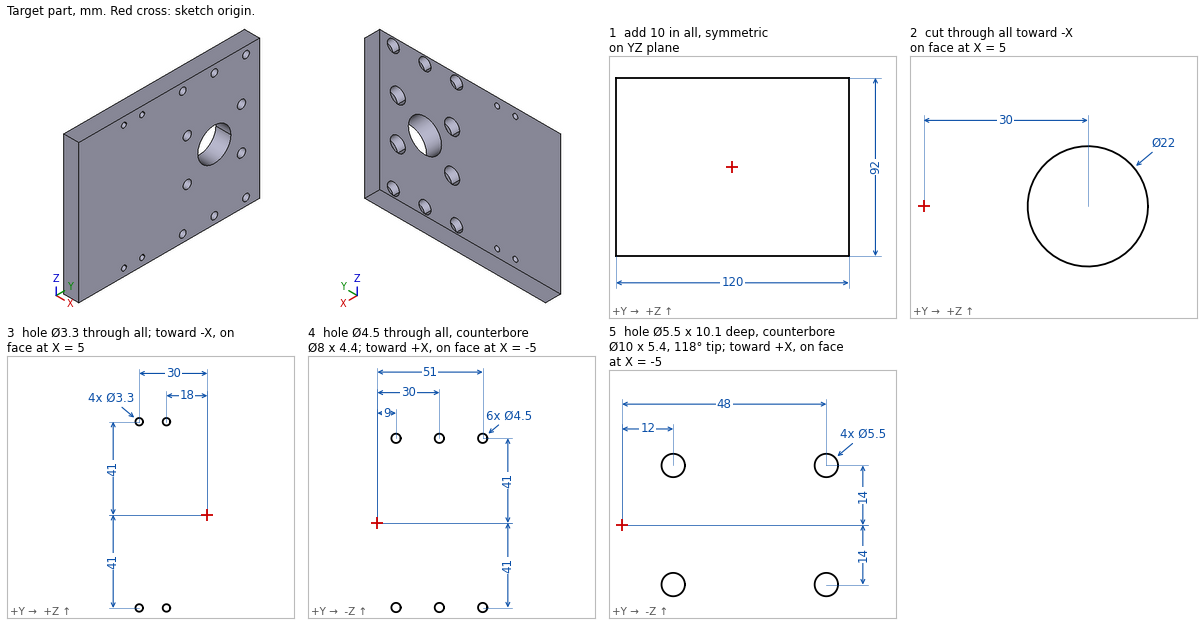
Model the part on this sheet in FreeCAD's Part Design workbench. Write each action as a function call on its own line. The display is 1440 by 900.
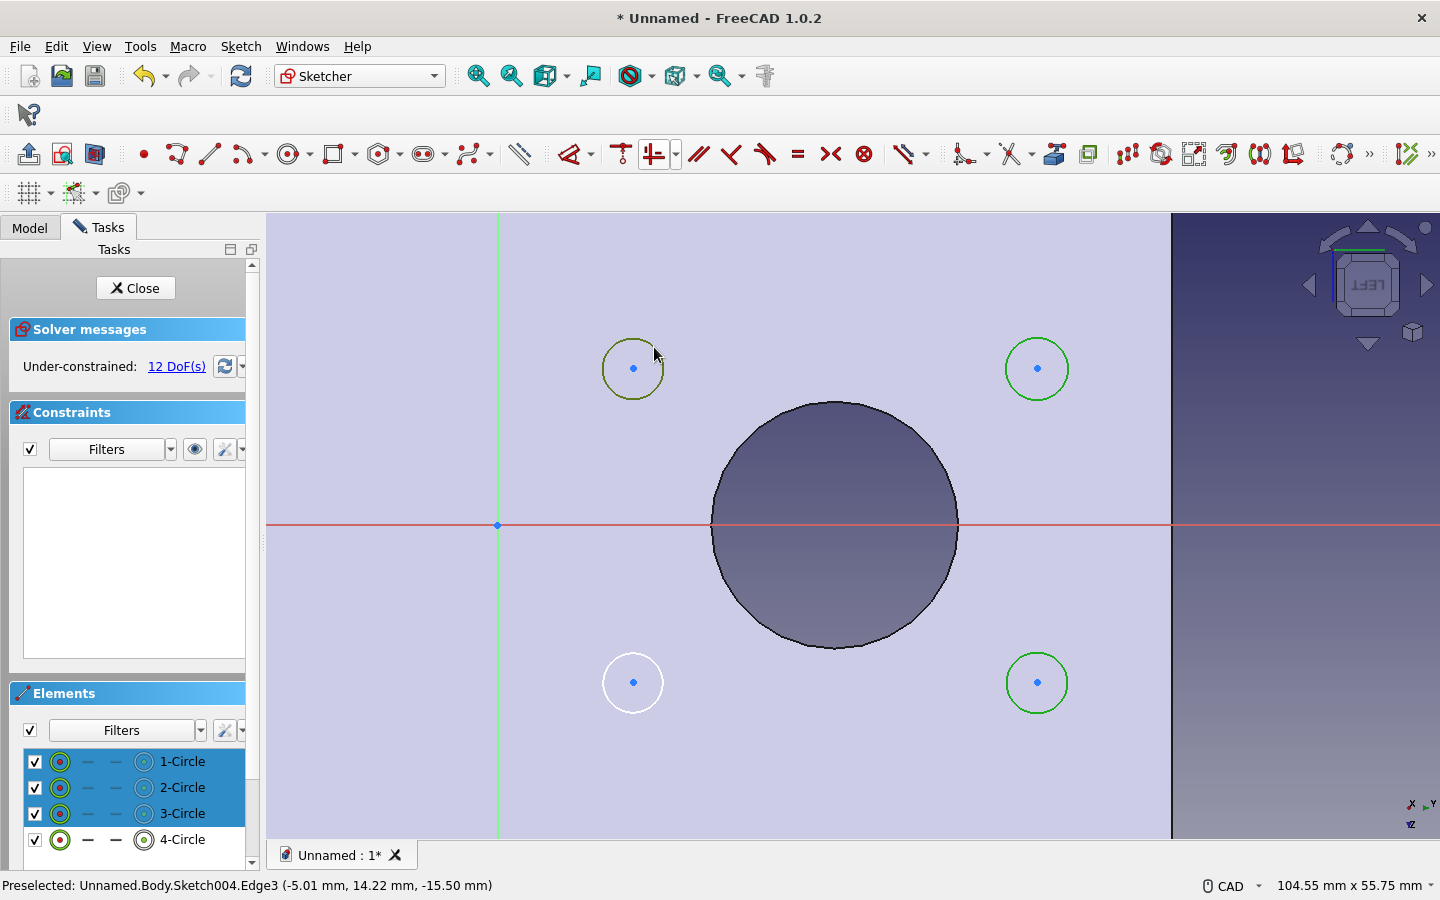
click(654, 662)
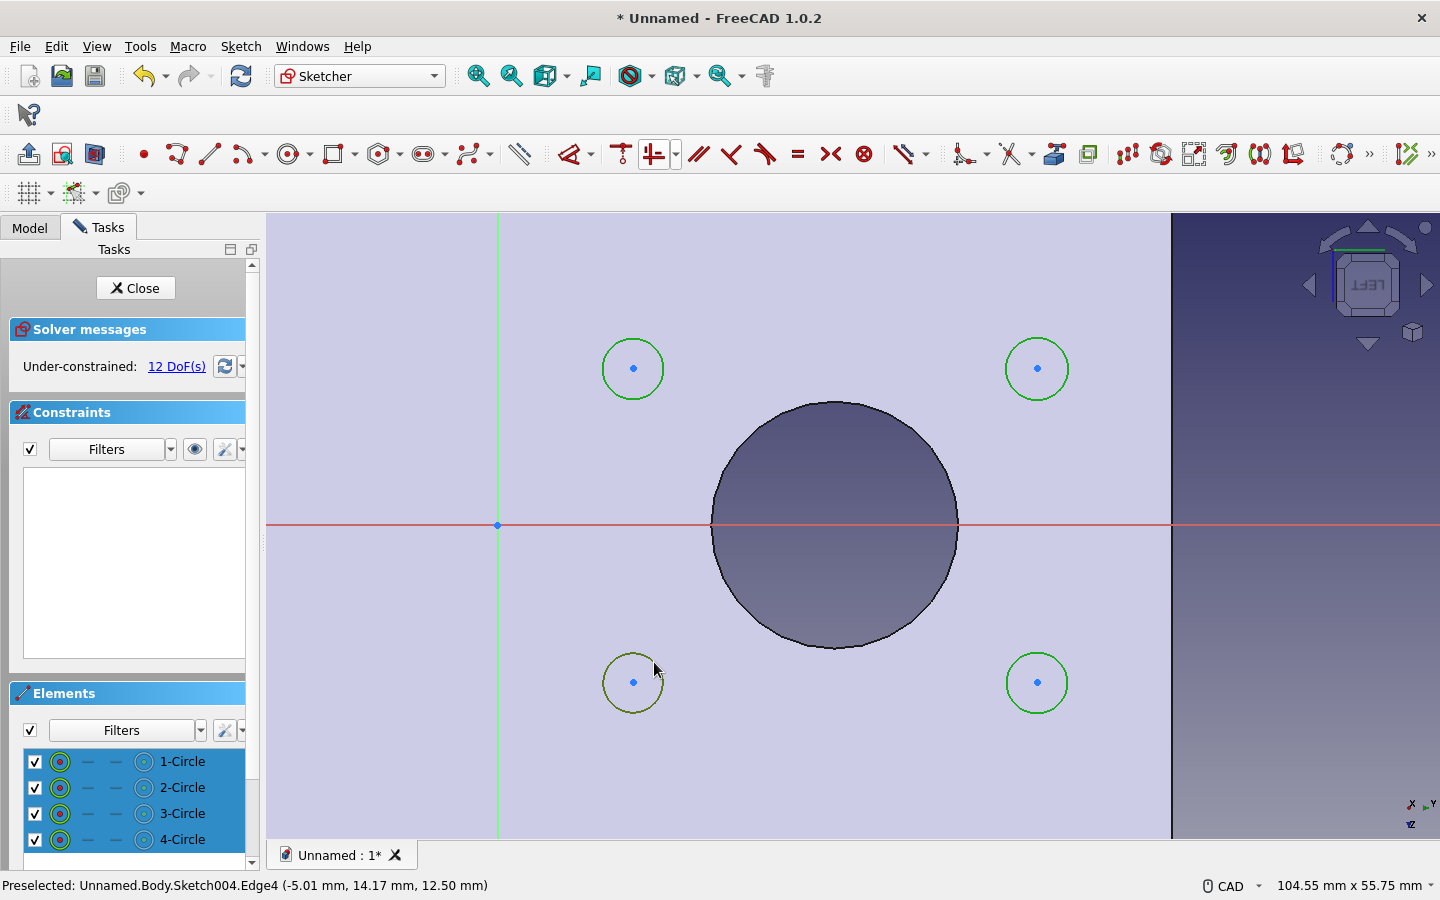
key(e)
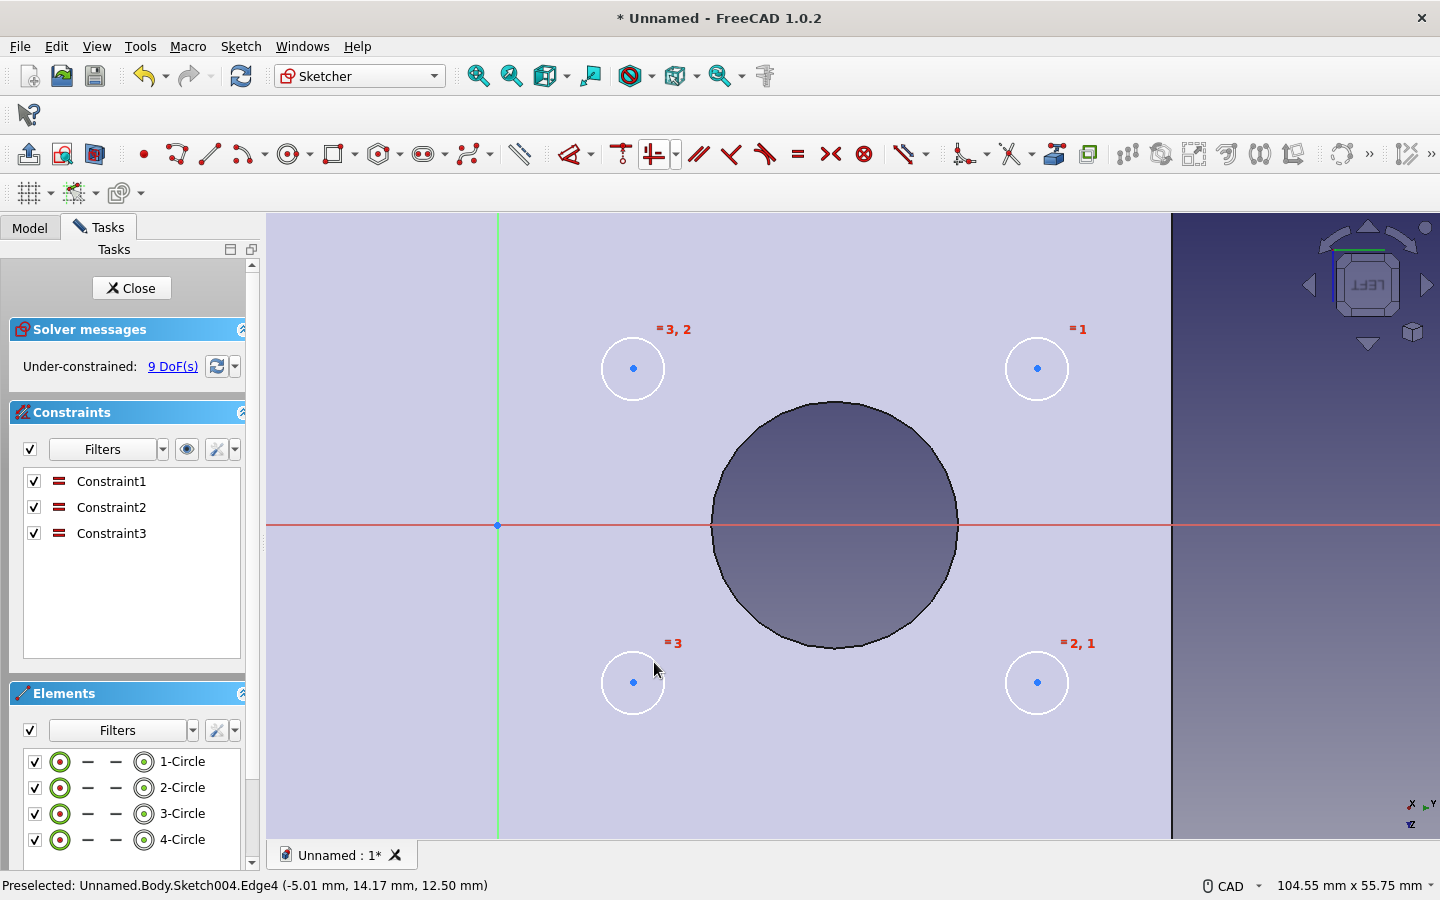
click(1037, 369)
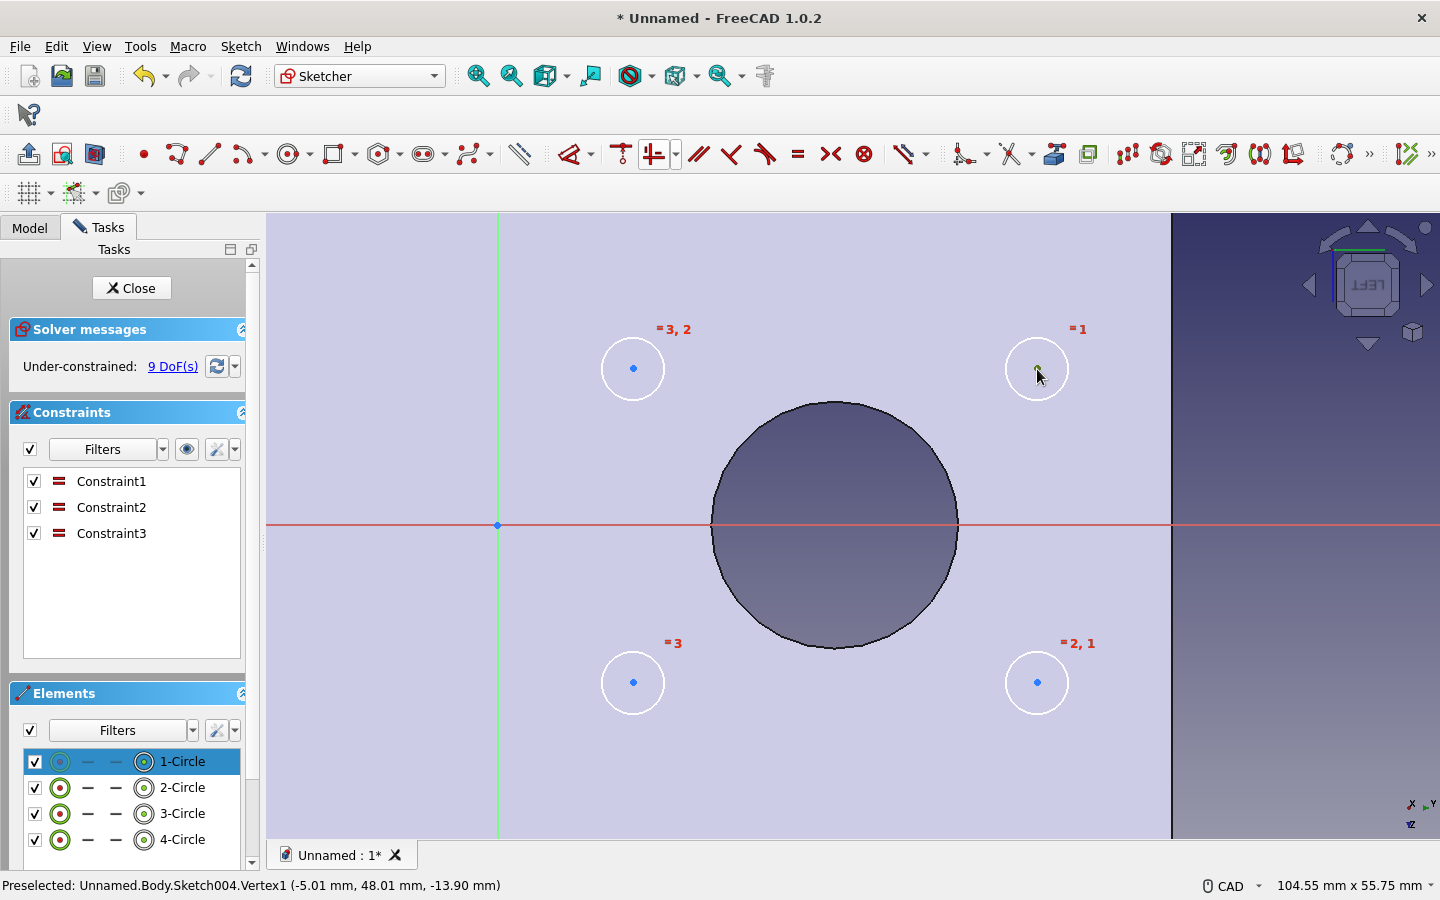
click(1037, 683)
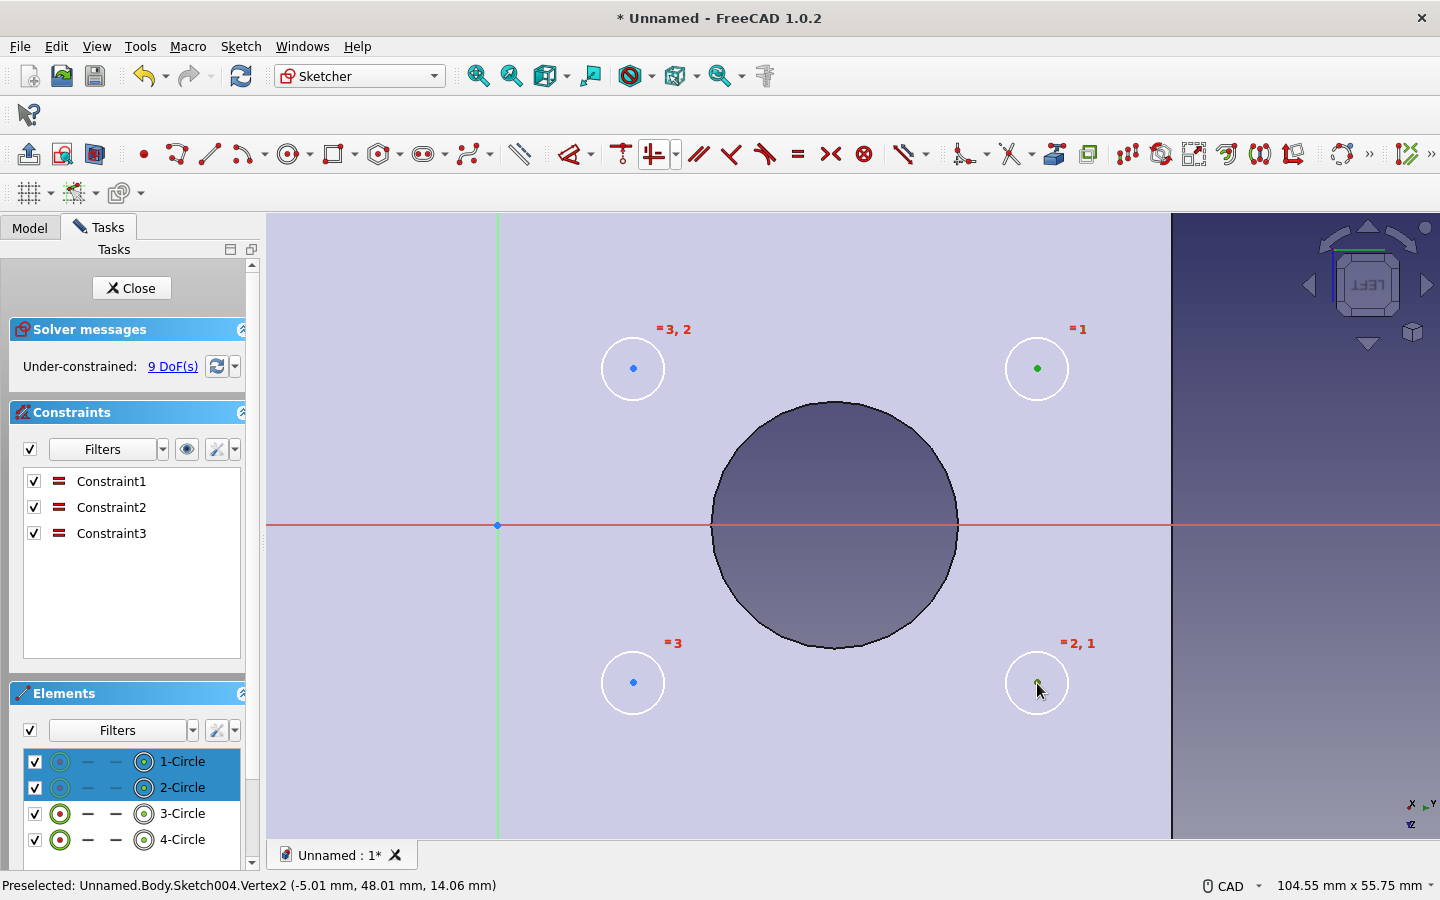
key(v)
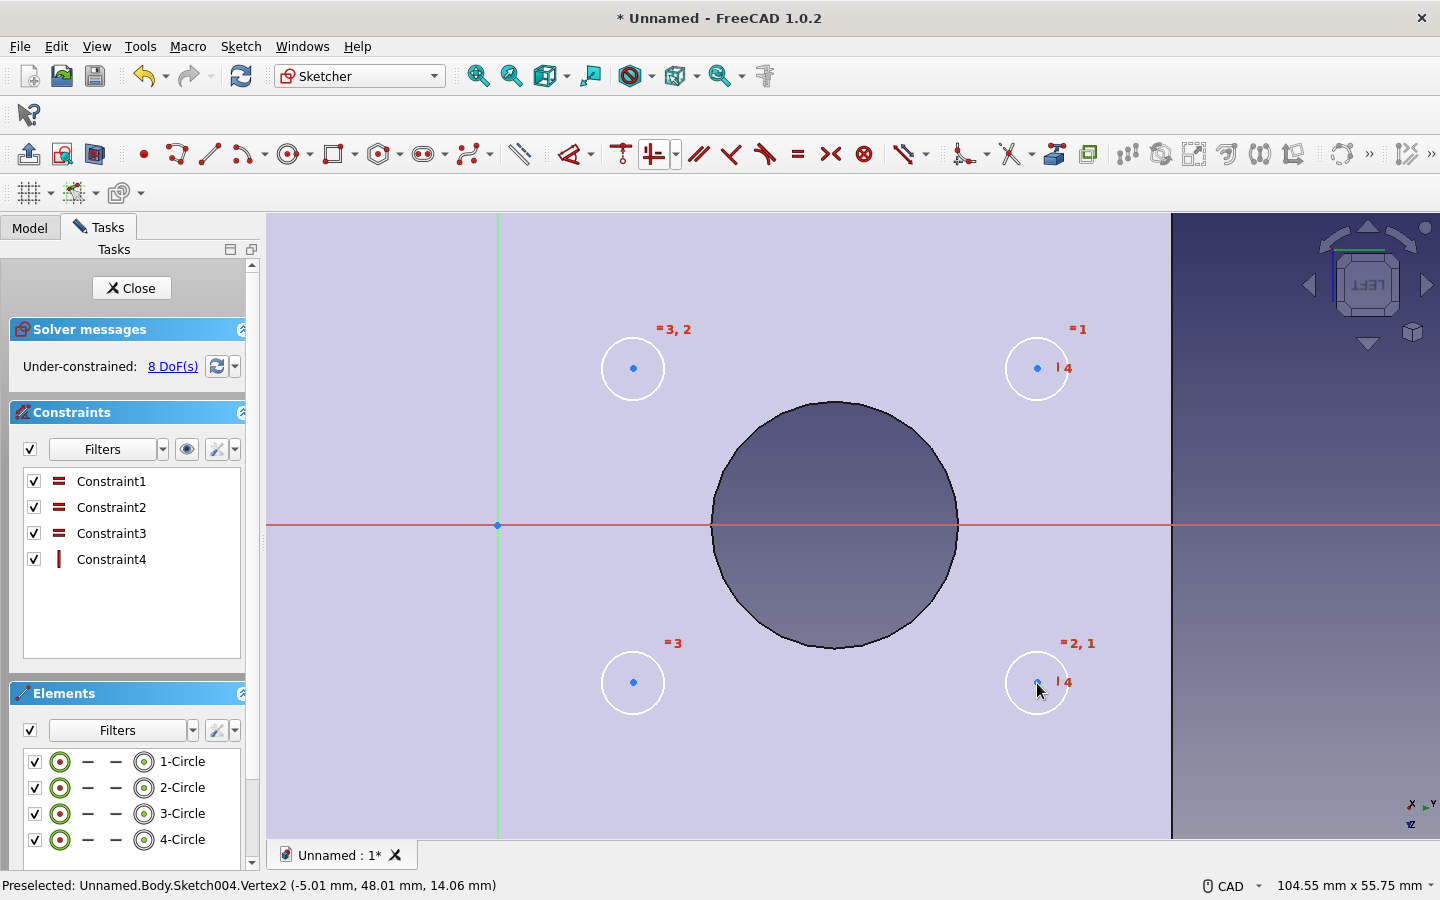
click(1037, 369)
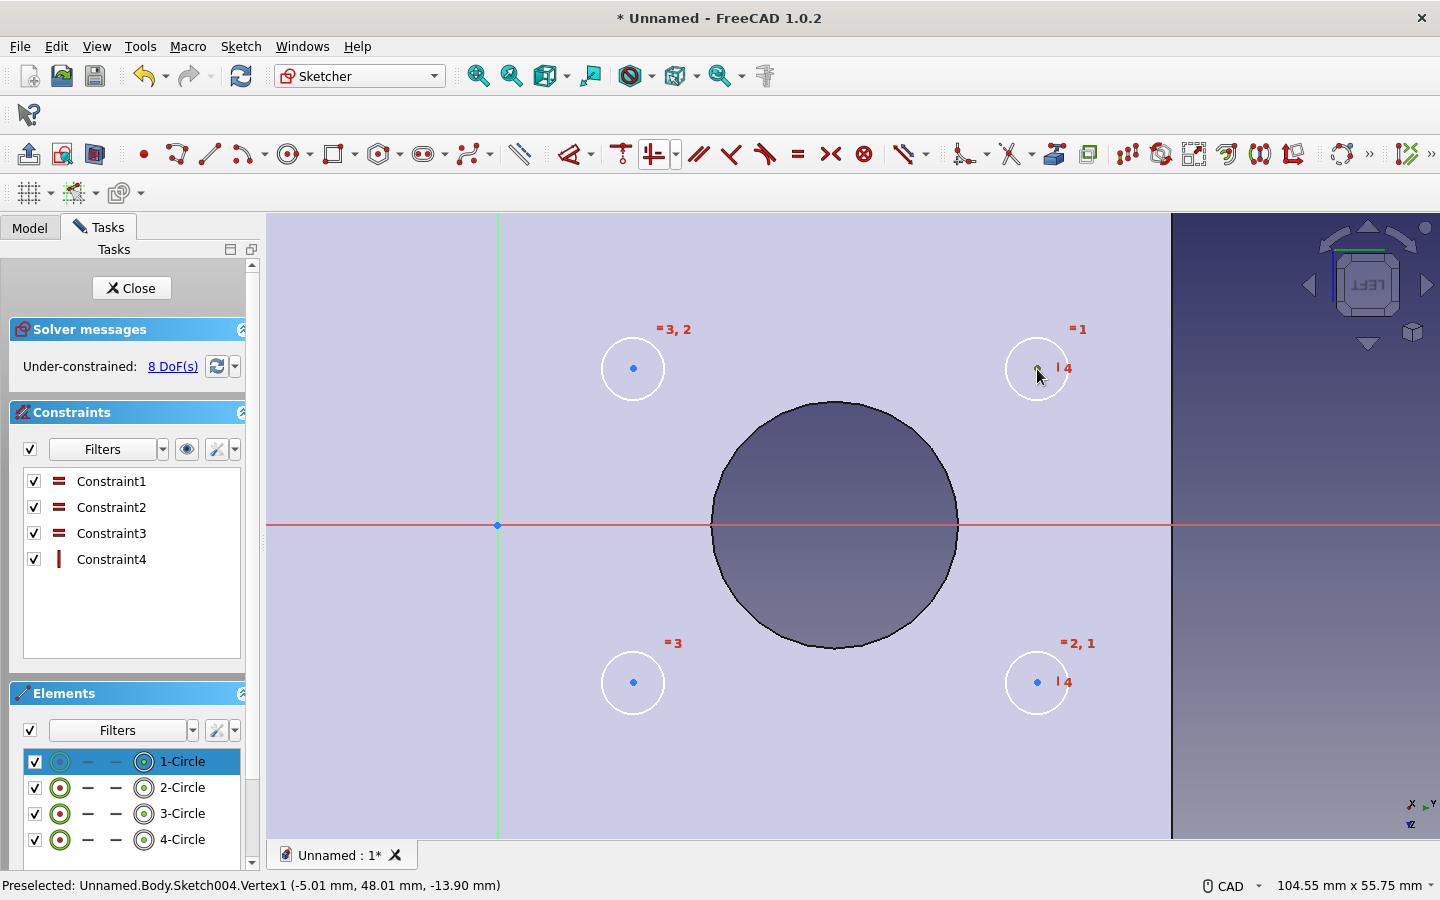
click(633, 369)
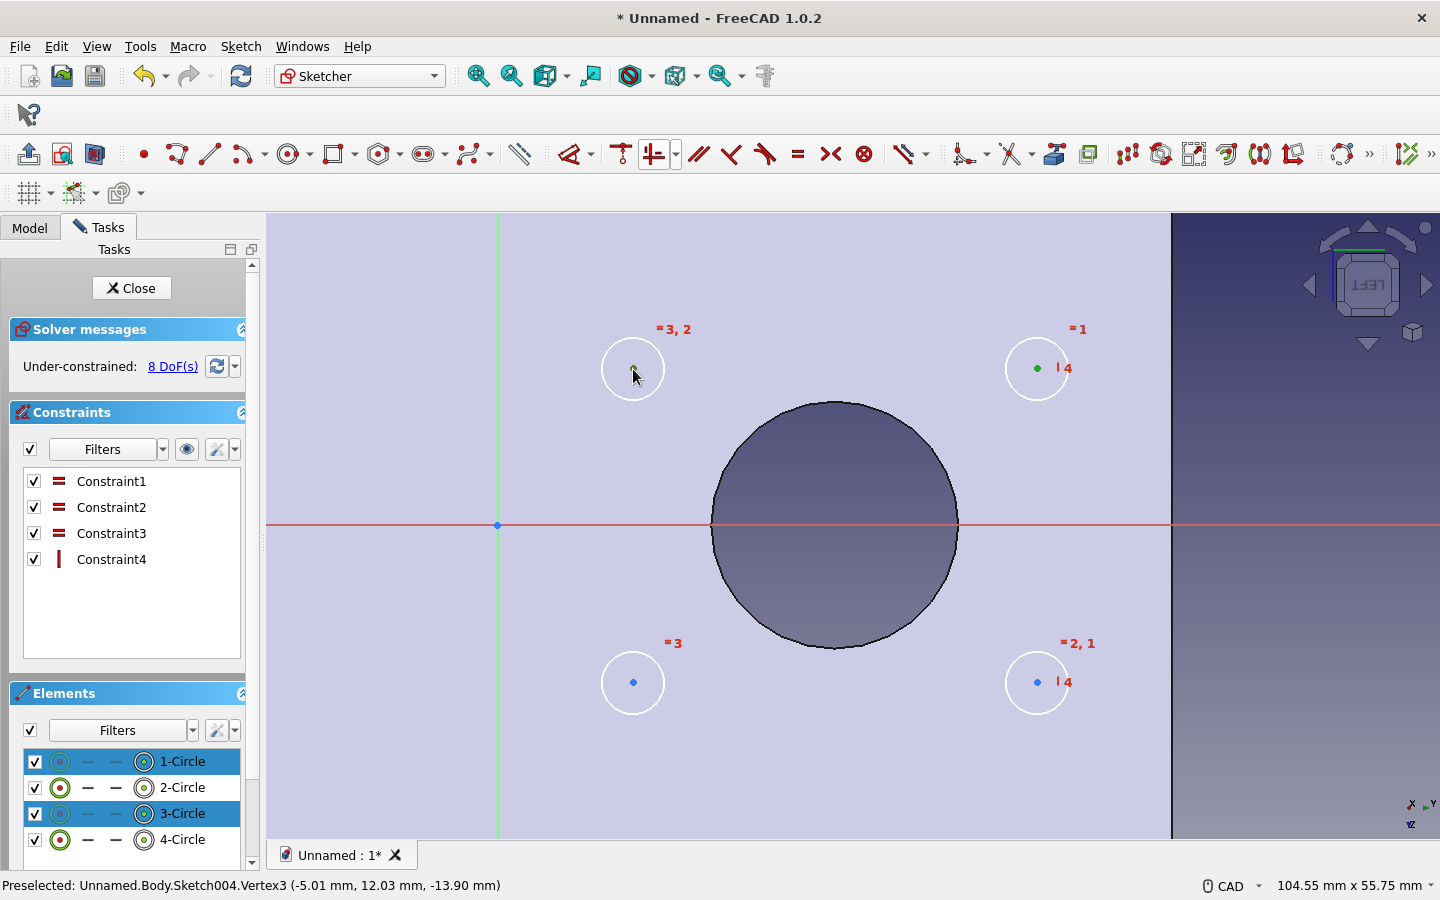
key(h)